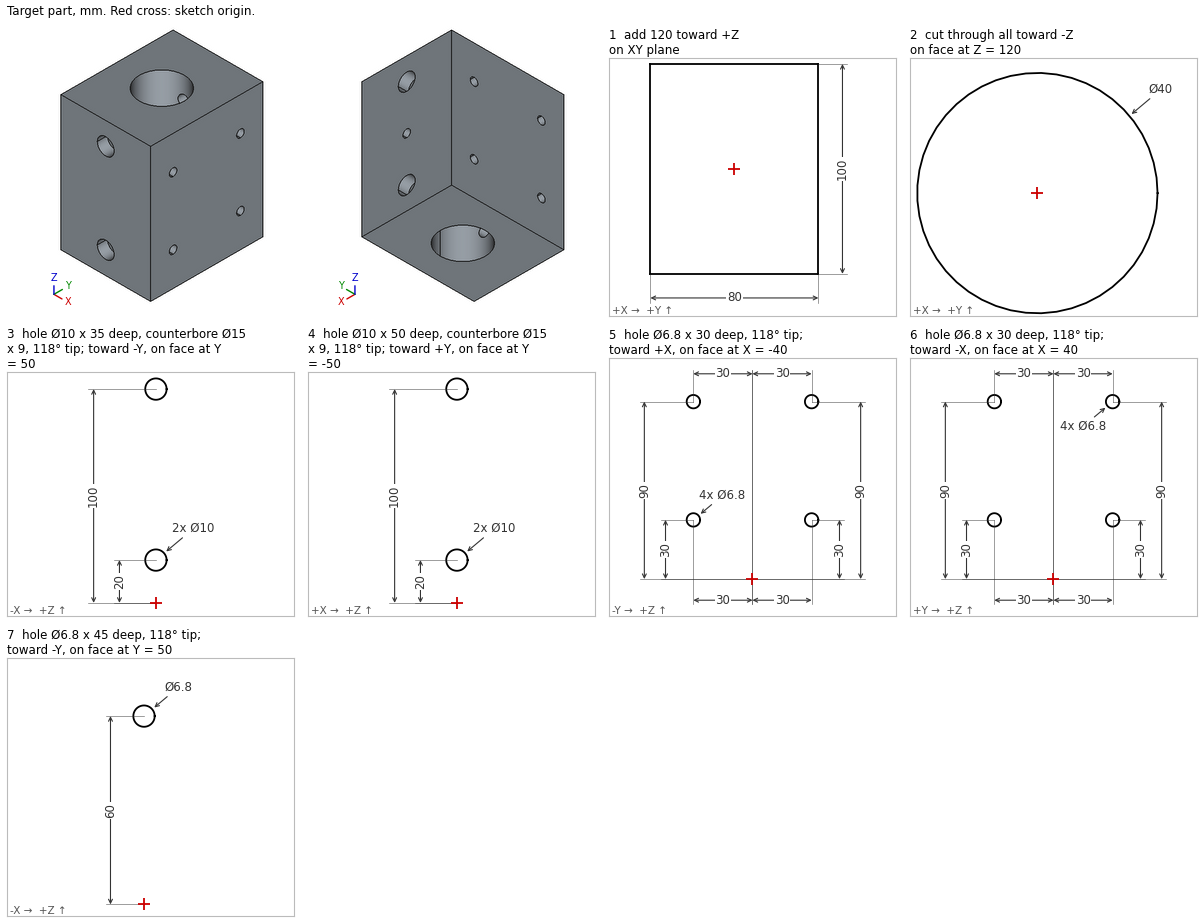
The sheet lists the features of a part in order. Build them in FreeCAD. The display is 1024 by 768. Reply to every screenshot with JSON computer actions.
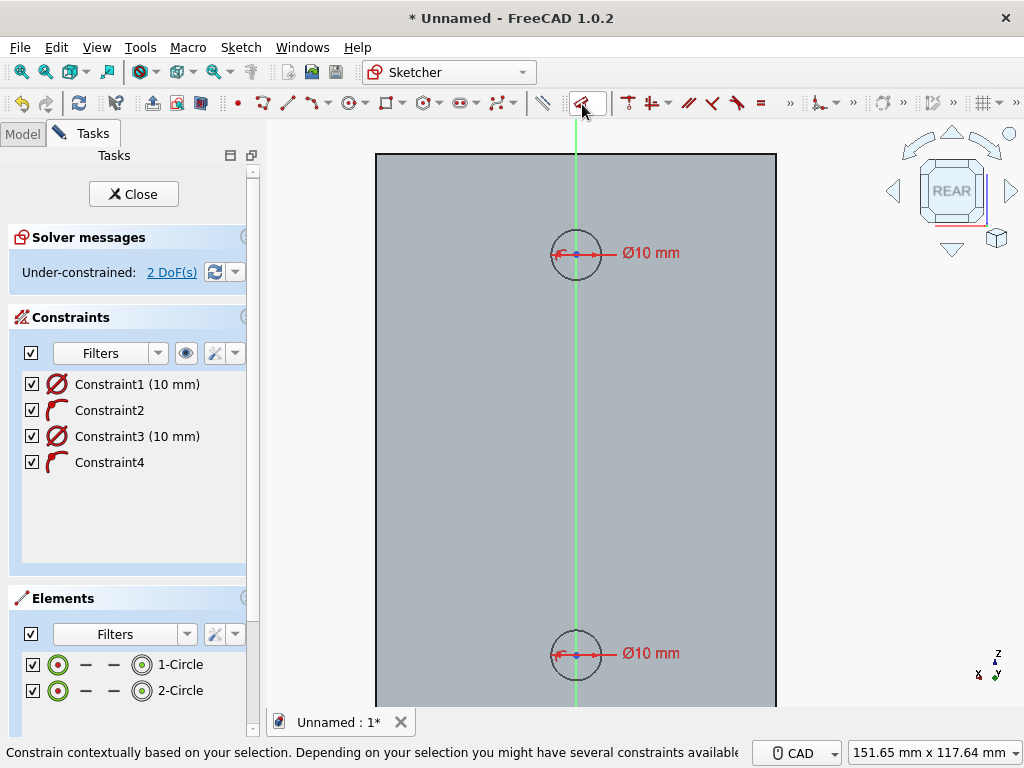
{"action": "left_click", "coordinate": [576, 655]}
{"action": "left_click", "coordinate": [610, 673]}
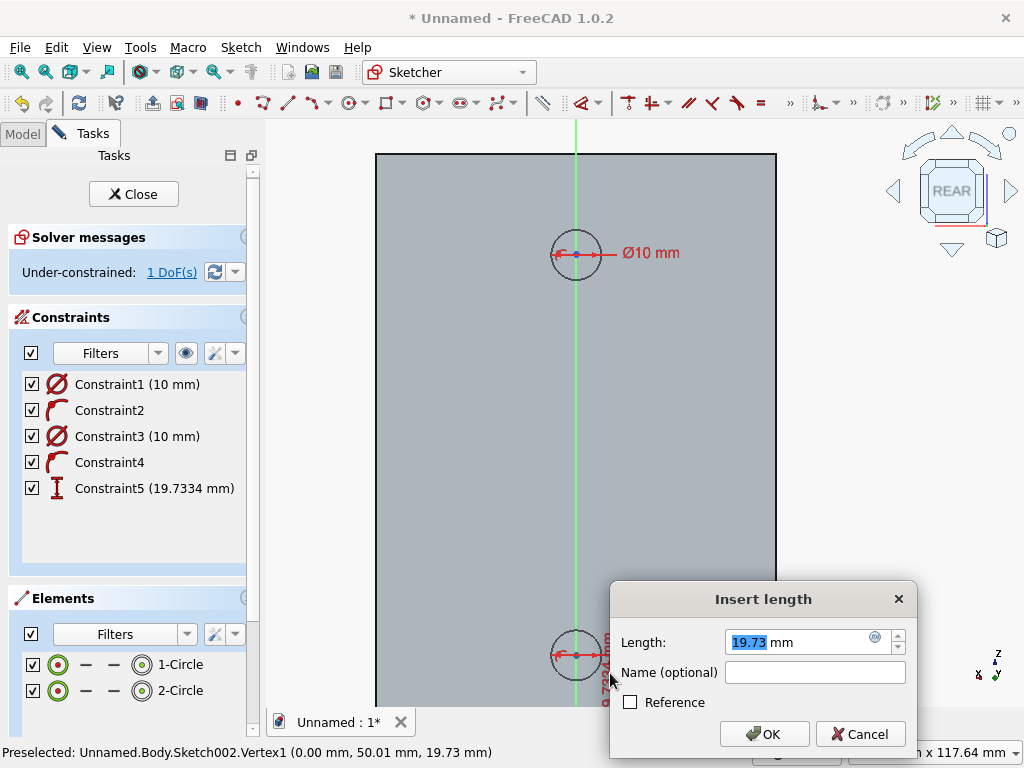
{"action": "type", "text": "20"}
{"action": "key", "text": "Return"}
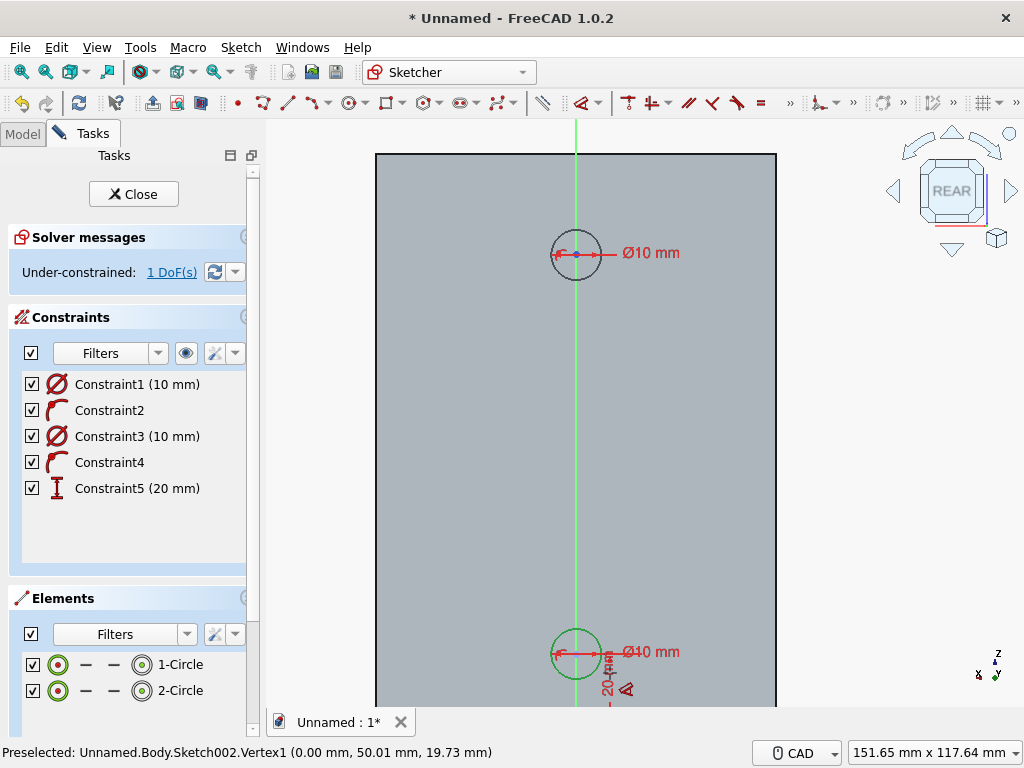
{"action": "left_click", "coordinate": [576, 255]}
{"action": "left_click", "coordinate": [610, 467]}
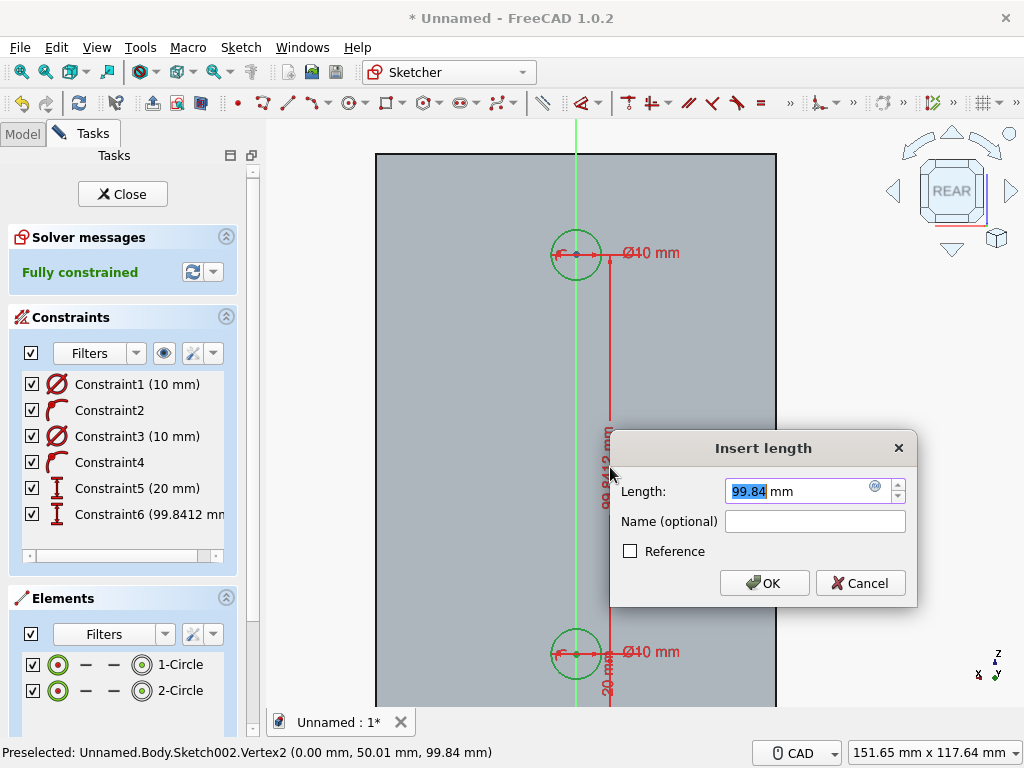
{"action": "type", "text": "100"}
{"action": "key", "text": "Return"}
{"action": "key", "text": "Escape"}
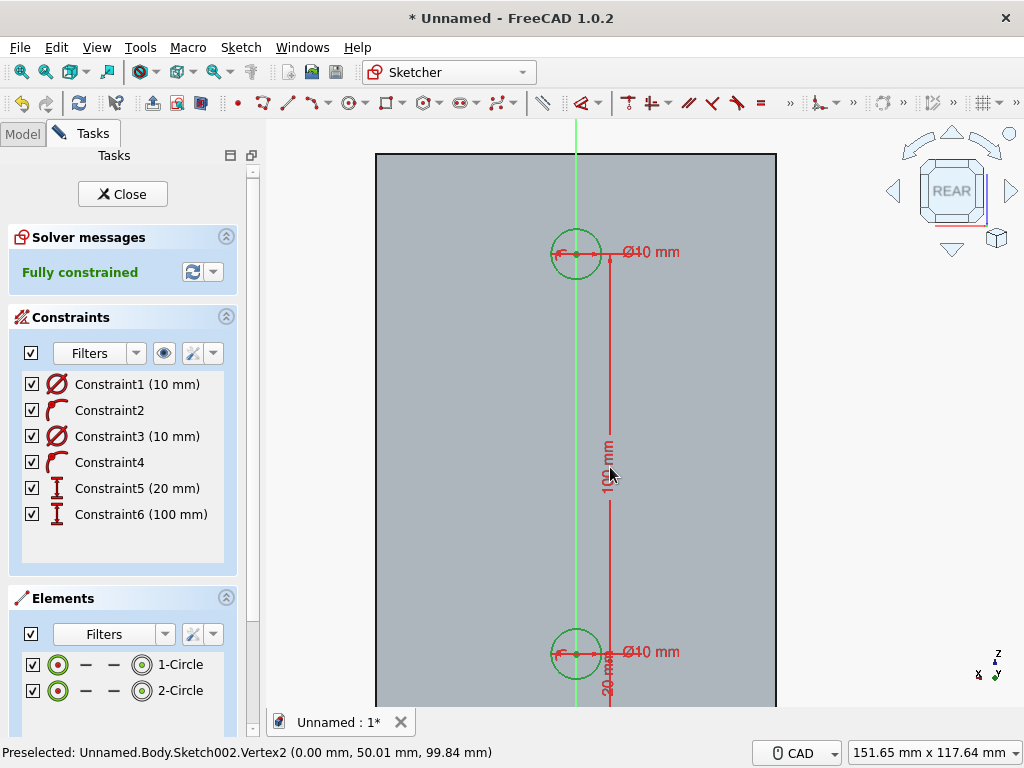
{"action": "left_click", "coordinate": [123, 194]}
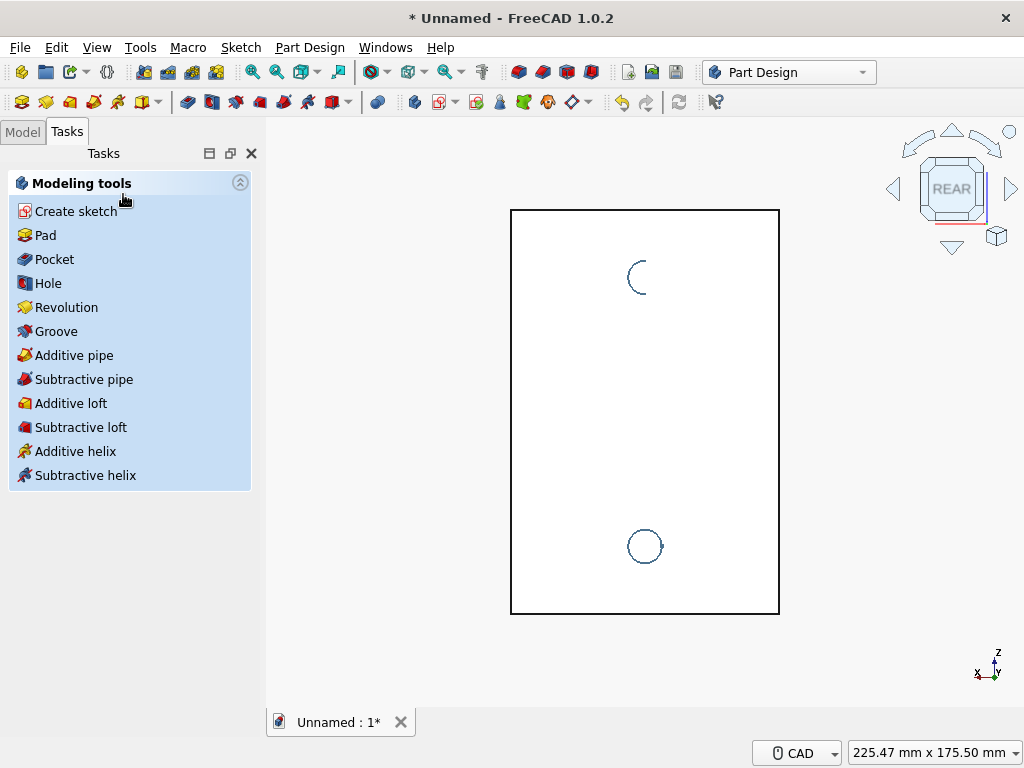
{"action": "left_click", "coordinate": [212, 102]}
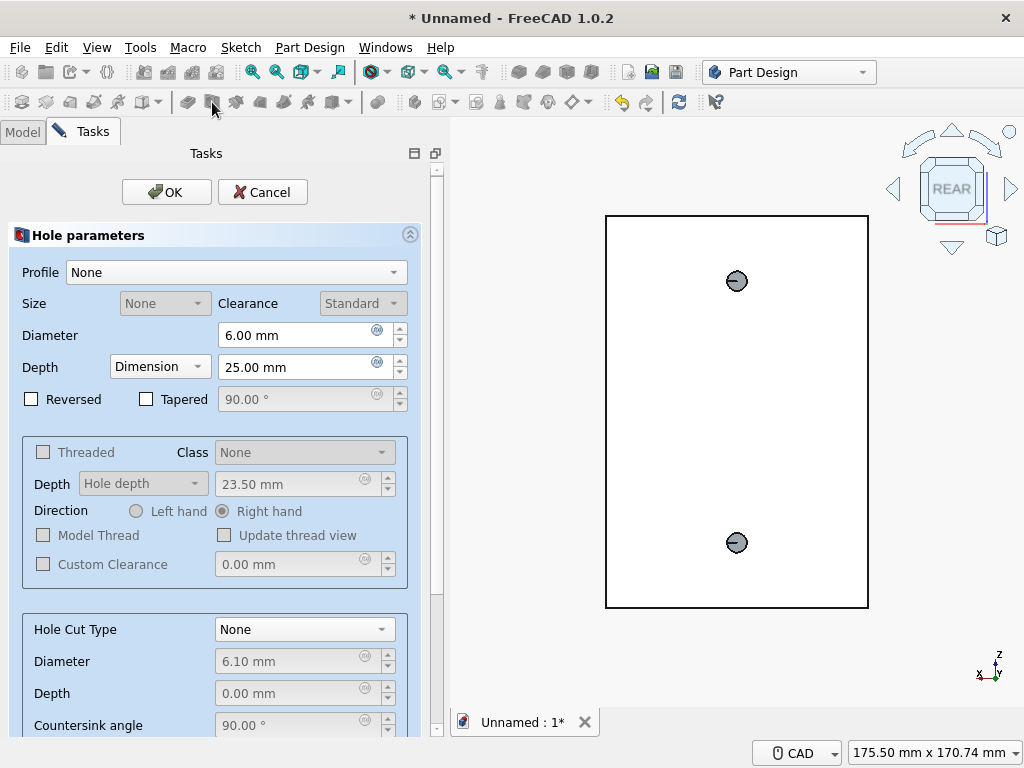
{"action": "triple_click", "coordinate": [305, 335]}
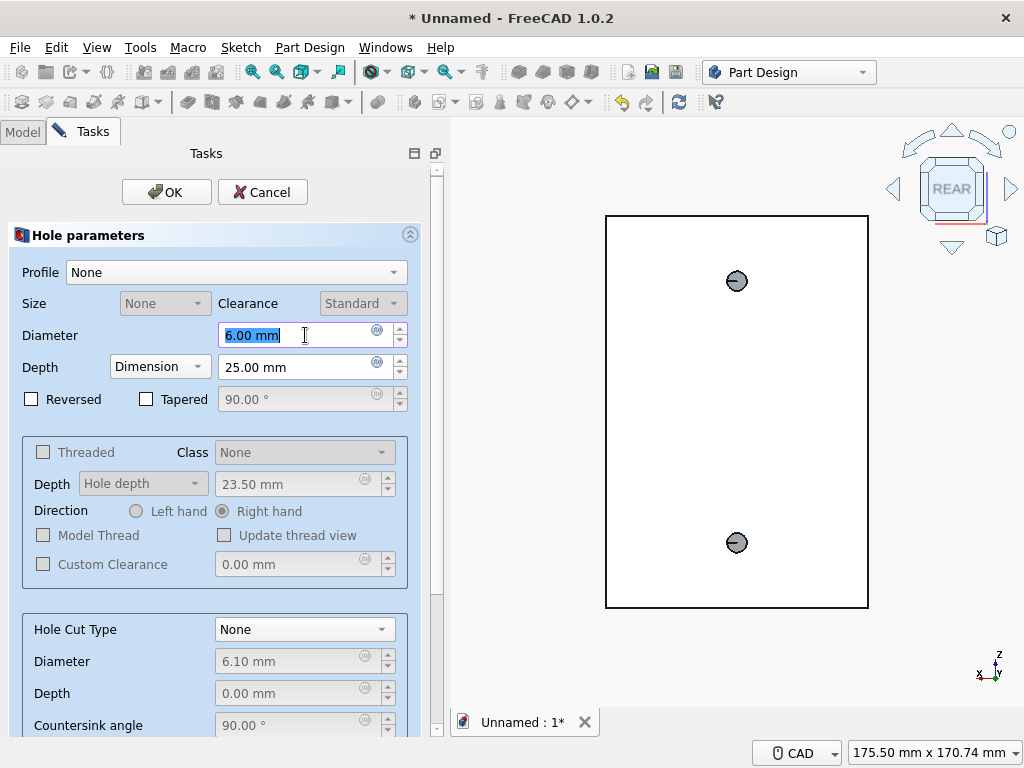
{"action": "type", "text": "10"}
{"action": "key", "text": "Tab"}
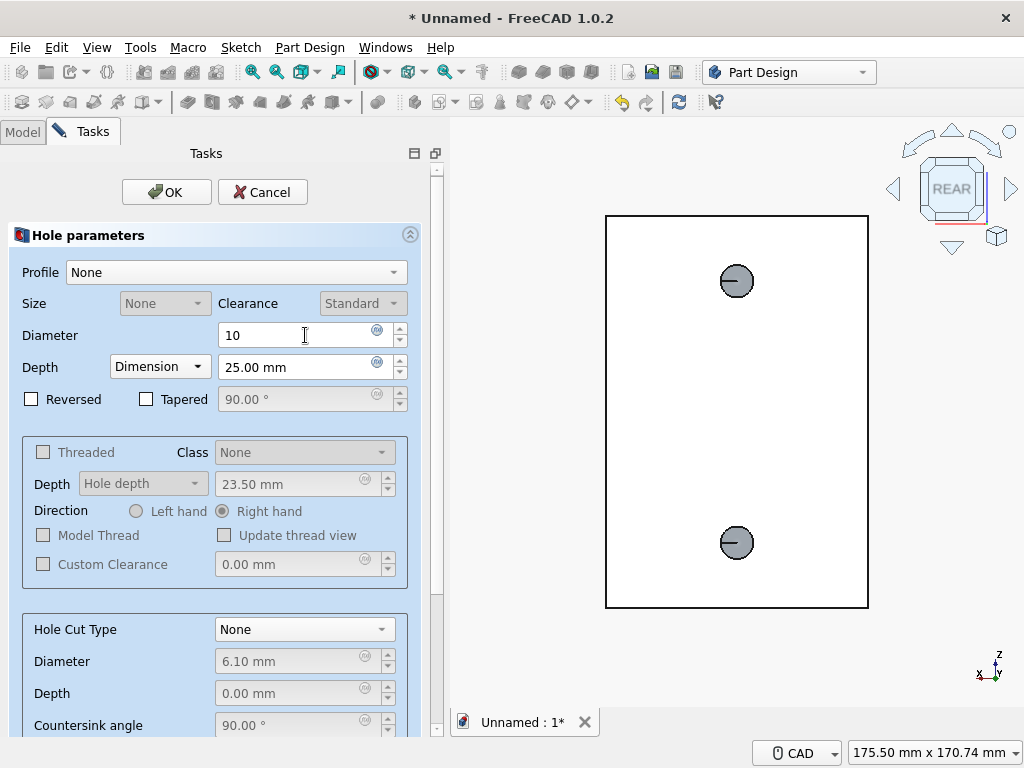
{"action": "triple_click", "coordinate": [305, 367]}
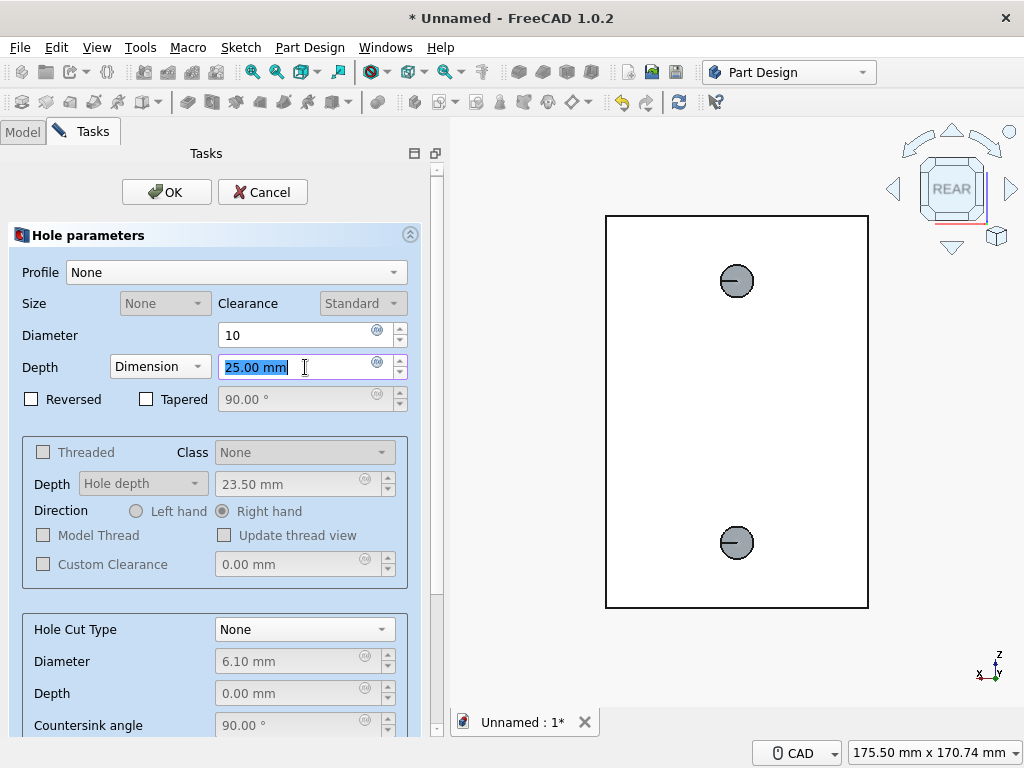
{"action": "type", "text": "35"}
{"action": "key", "text": "Tab"}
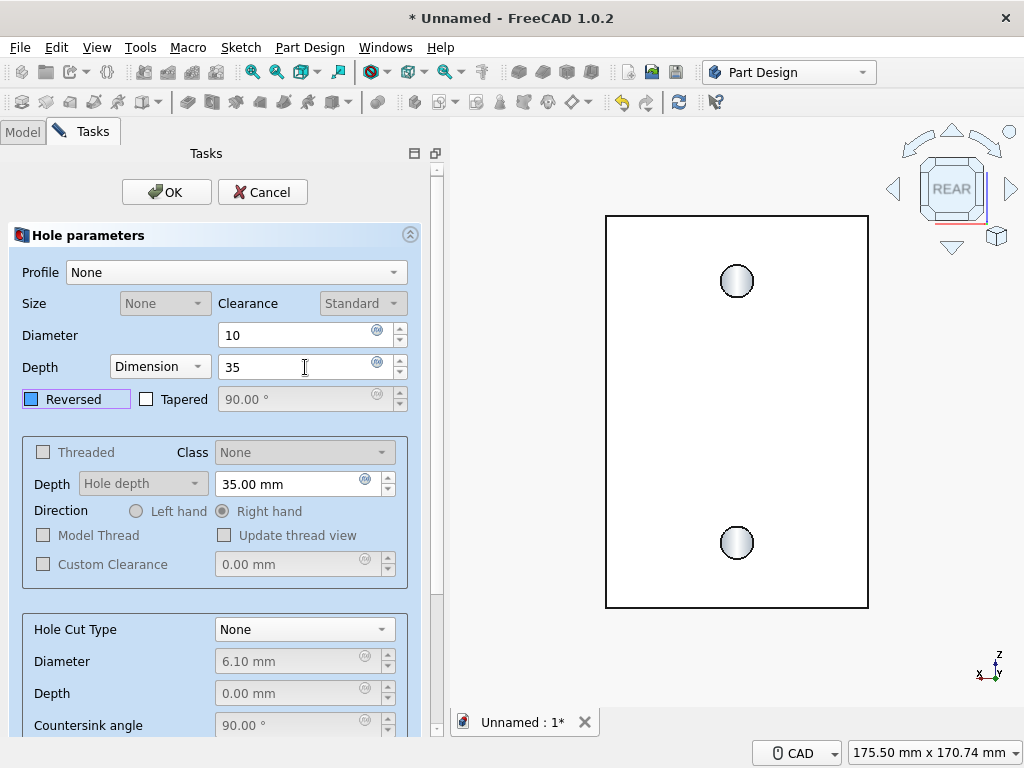
{"action": "left_click", "coordinate": [306, 630]}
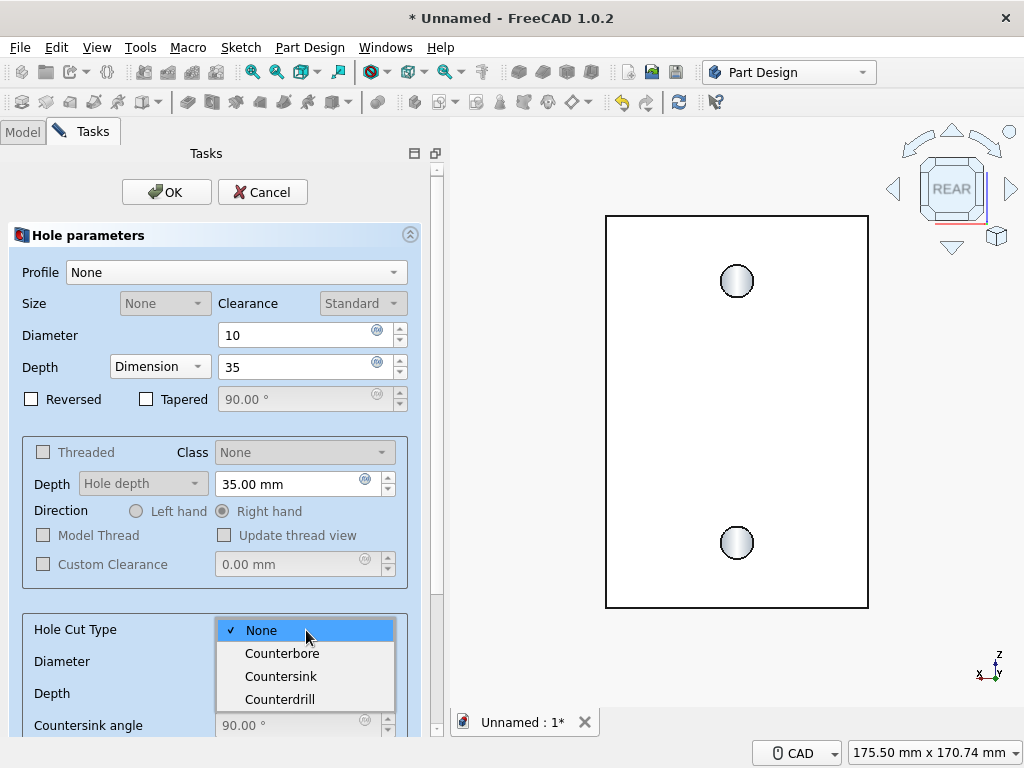
{"action": "left_click", "coordinate": [304, 654]}